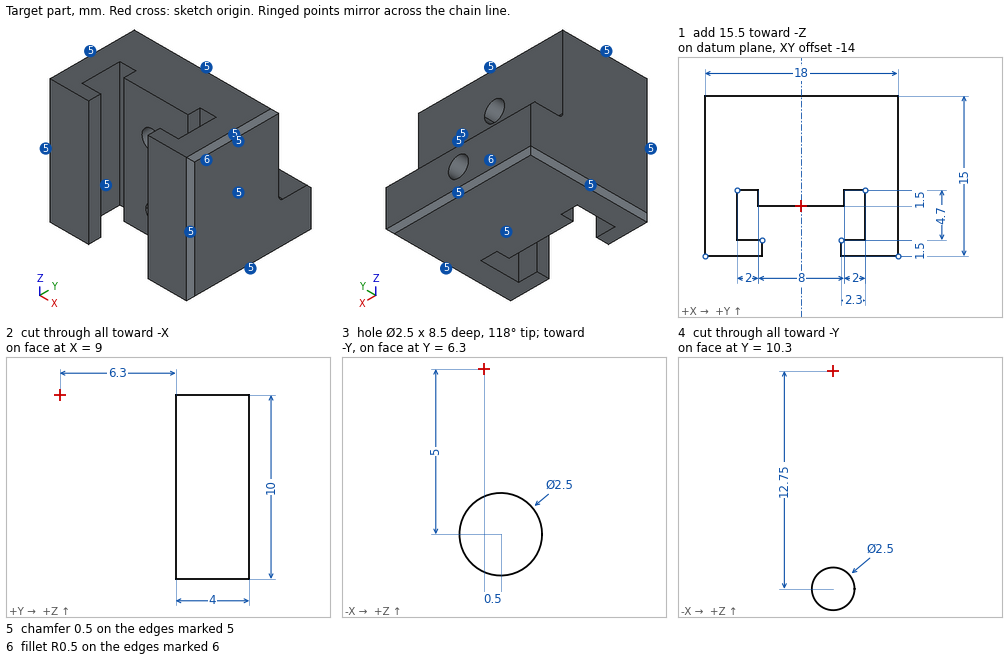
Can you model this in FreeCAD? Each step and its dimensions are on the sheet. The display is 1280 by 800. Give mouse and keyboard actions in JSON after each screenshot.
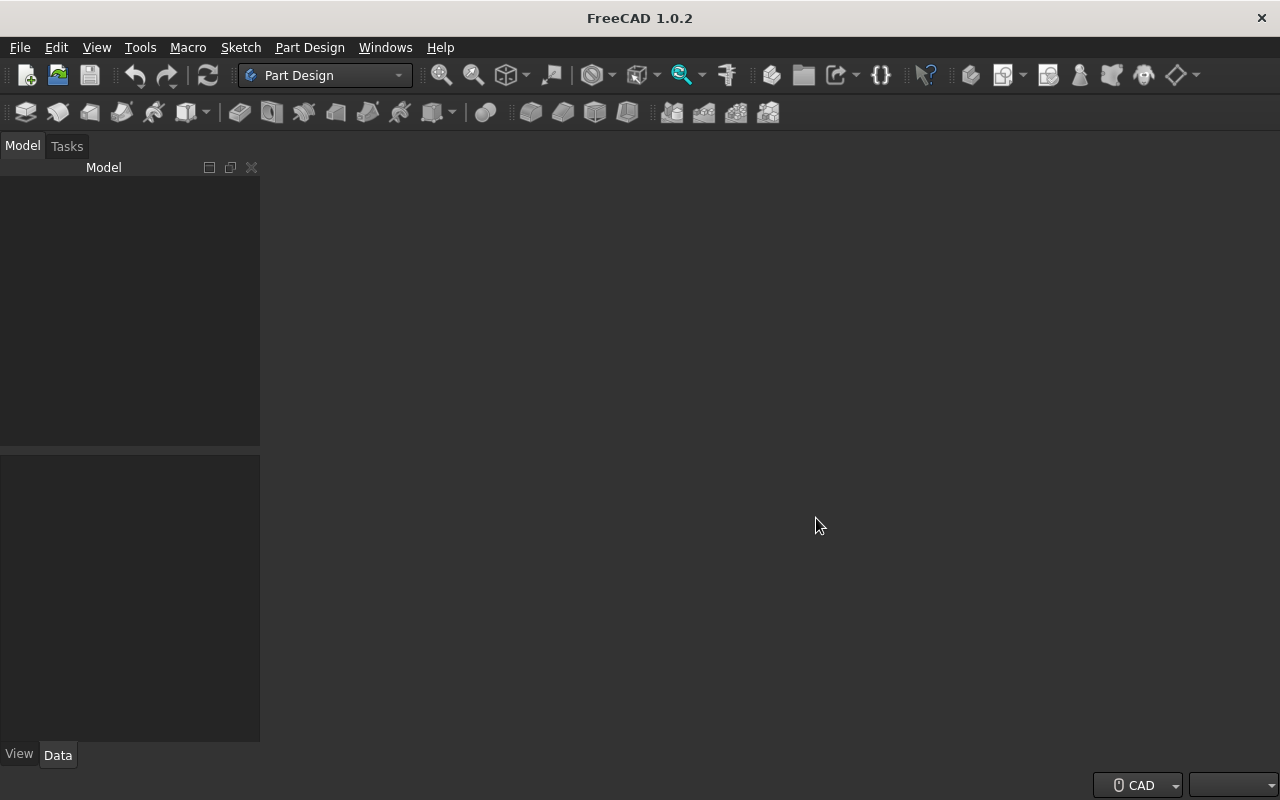
{"action": "left_click", "coordinate": [26, 76]}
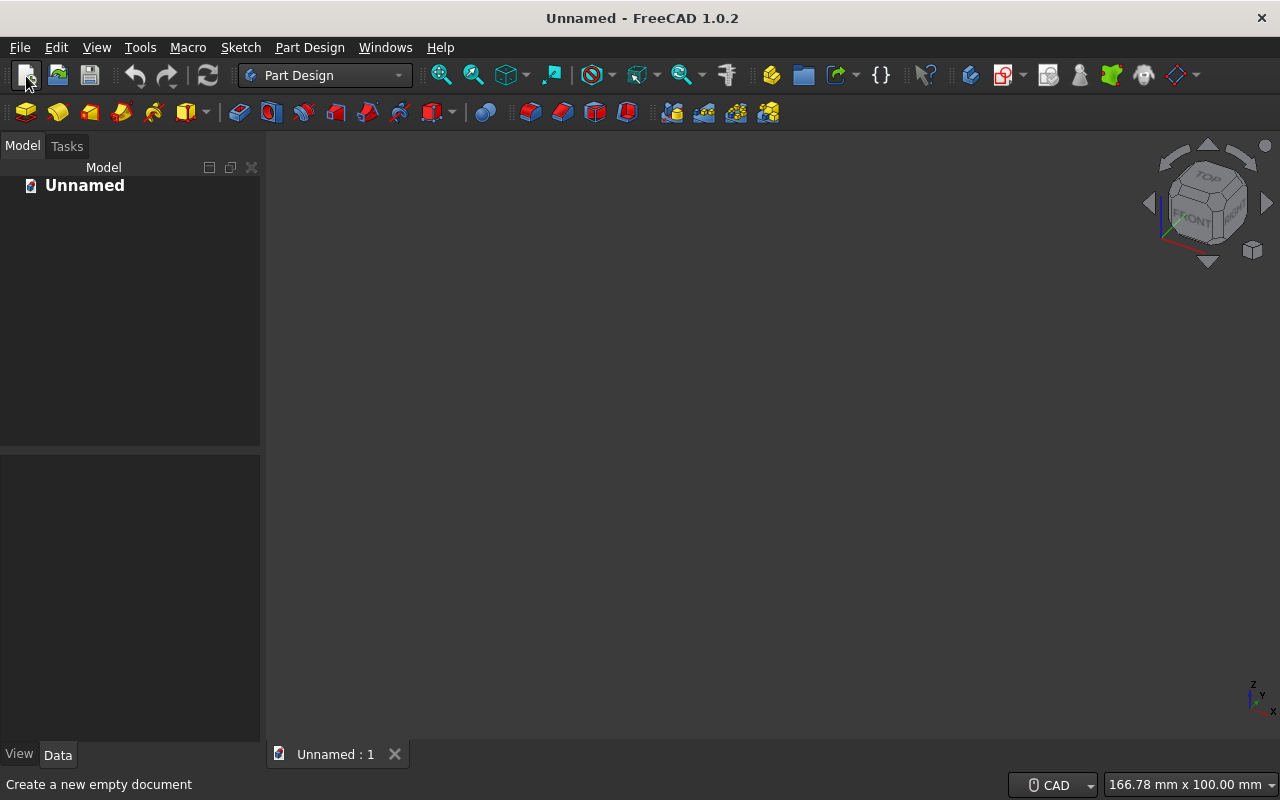
{"action": "left_click", "coordinate": [972, 76]}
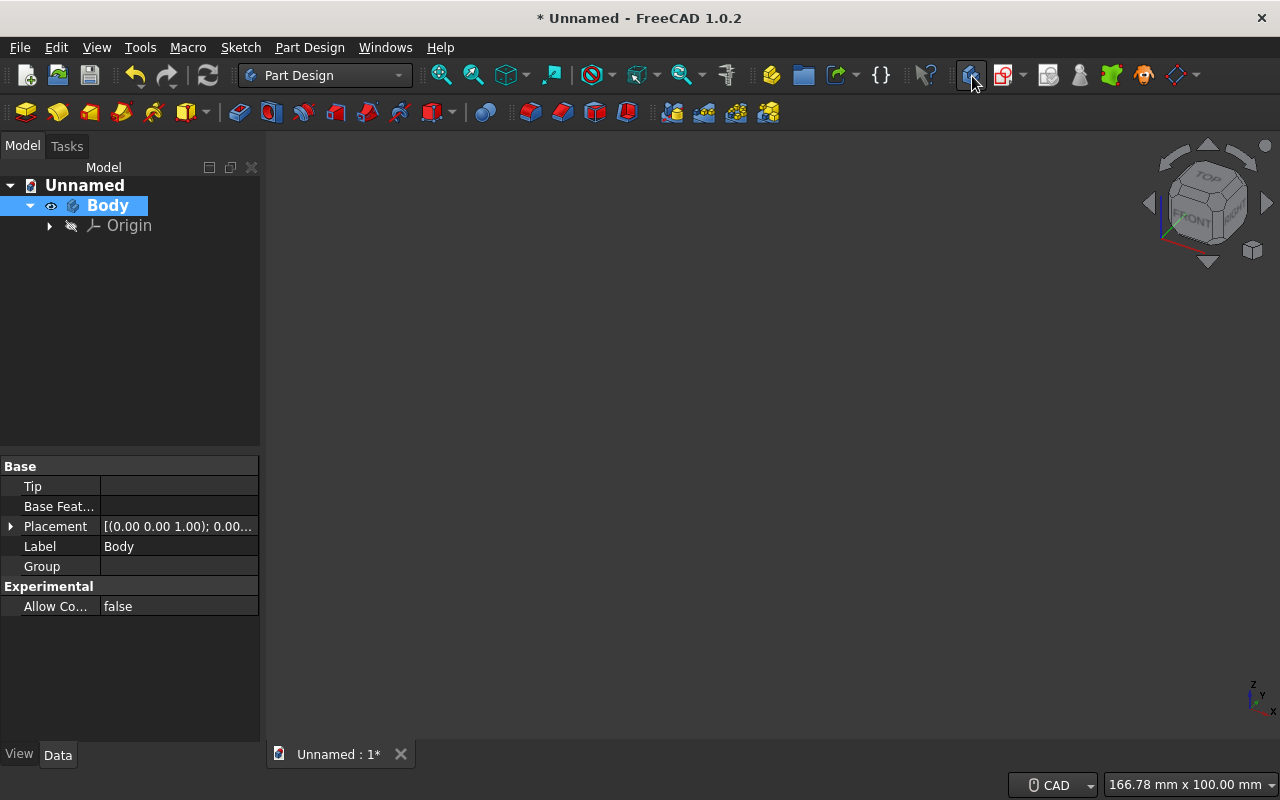
{"action": "left_click", "coordinate": [50, 226]}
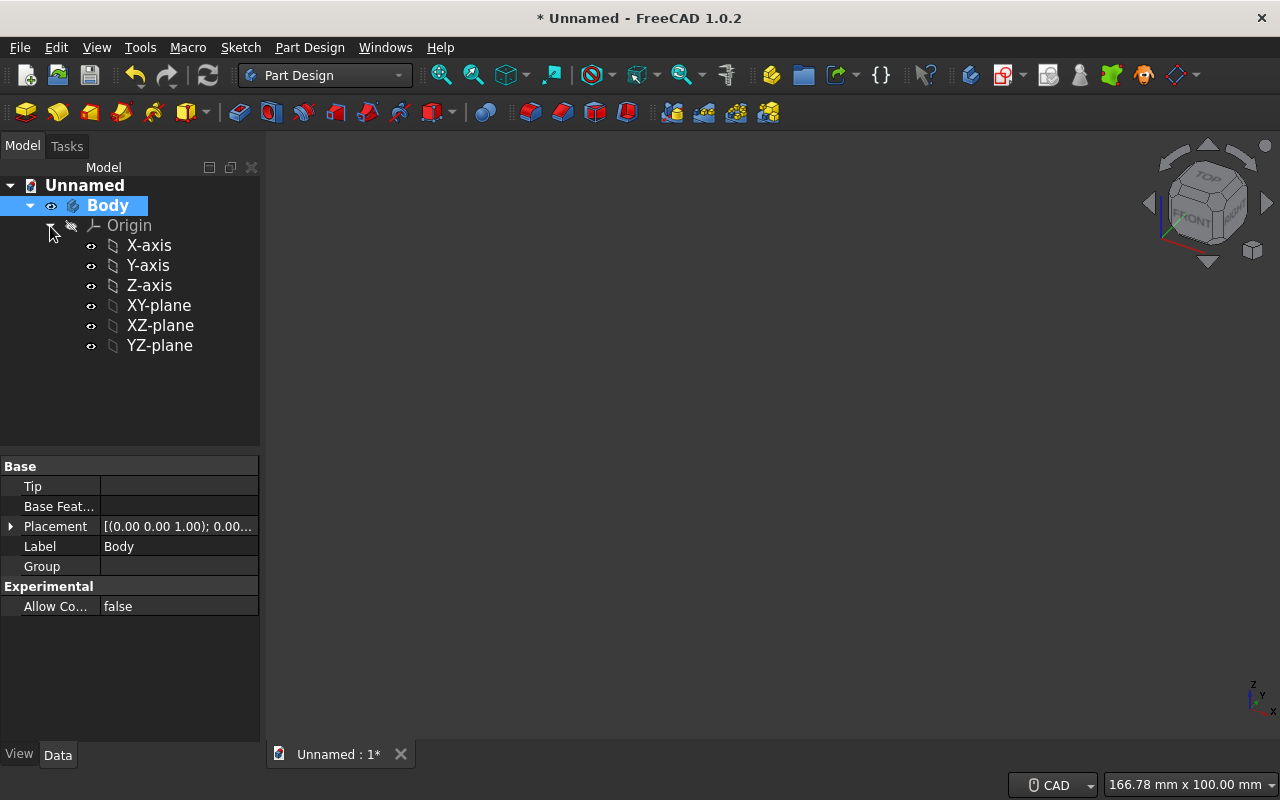
{"action": "left_click", "coordinate": [136, 306]}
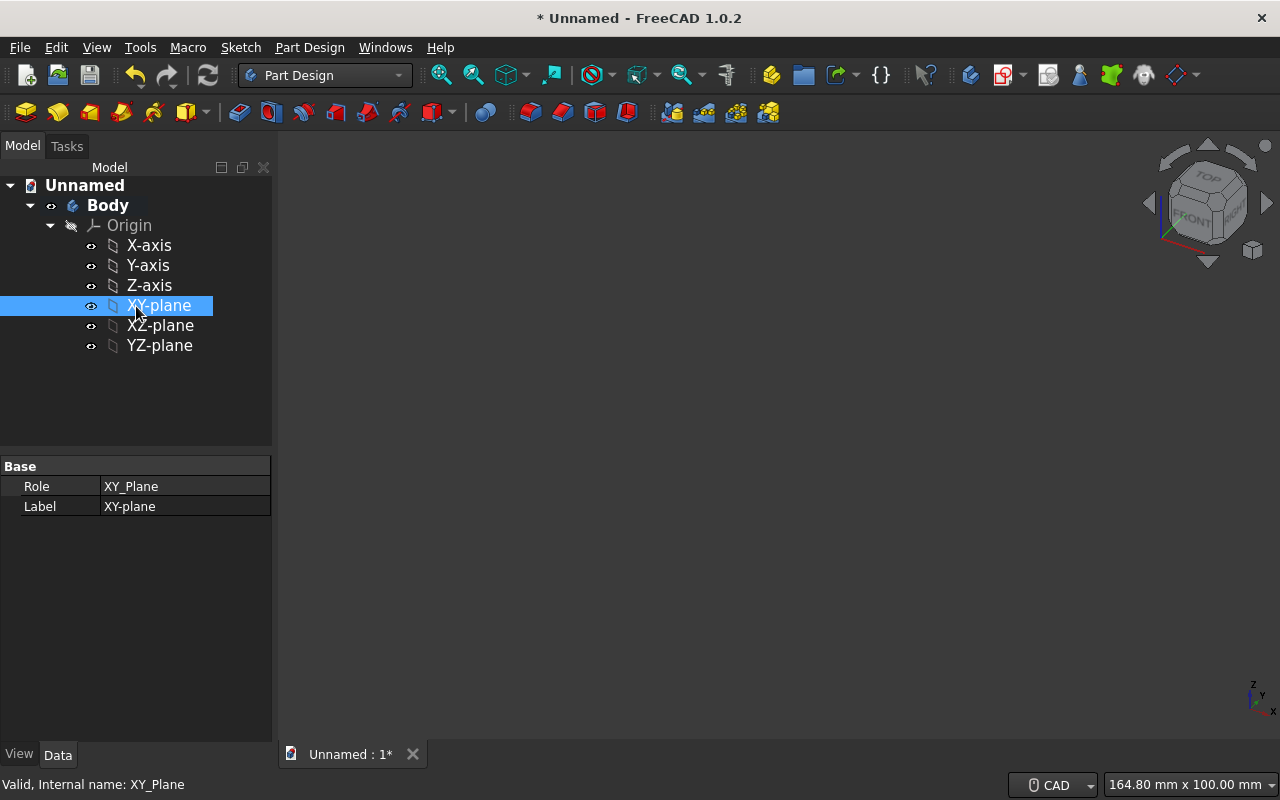
{"action": "left_click", "coordinate": [1176, 76]}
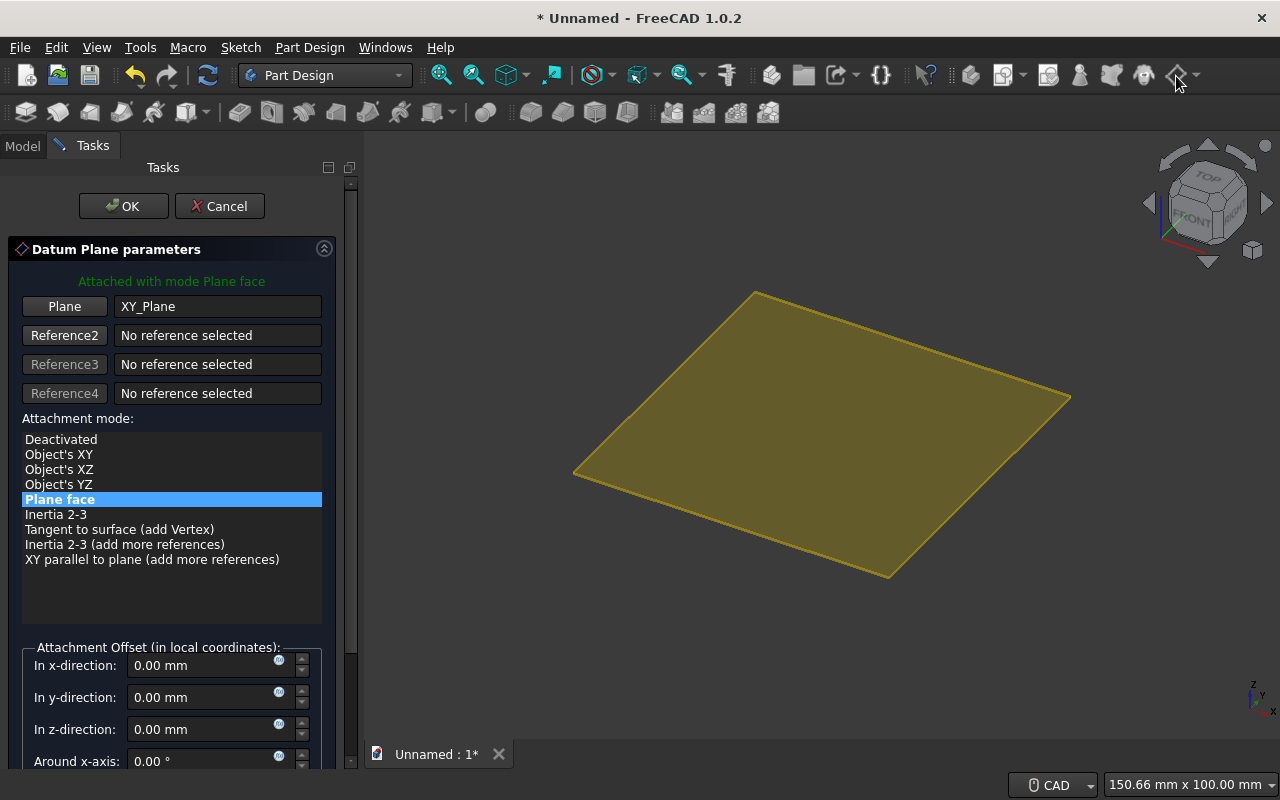
{"action": "triple_click", "coordinate": [210, 729]}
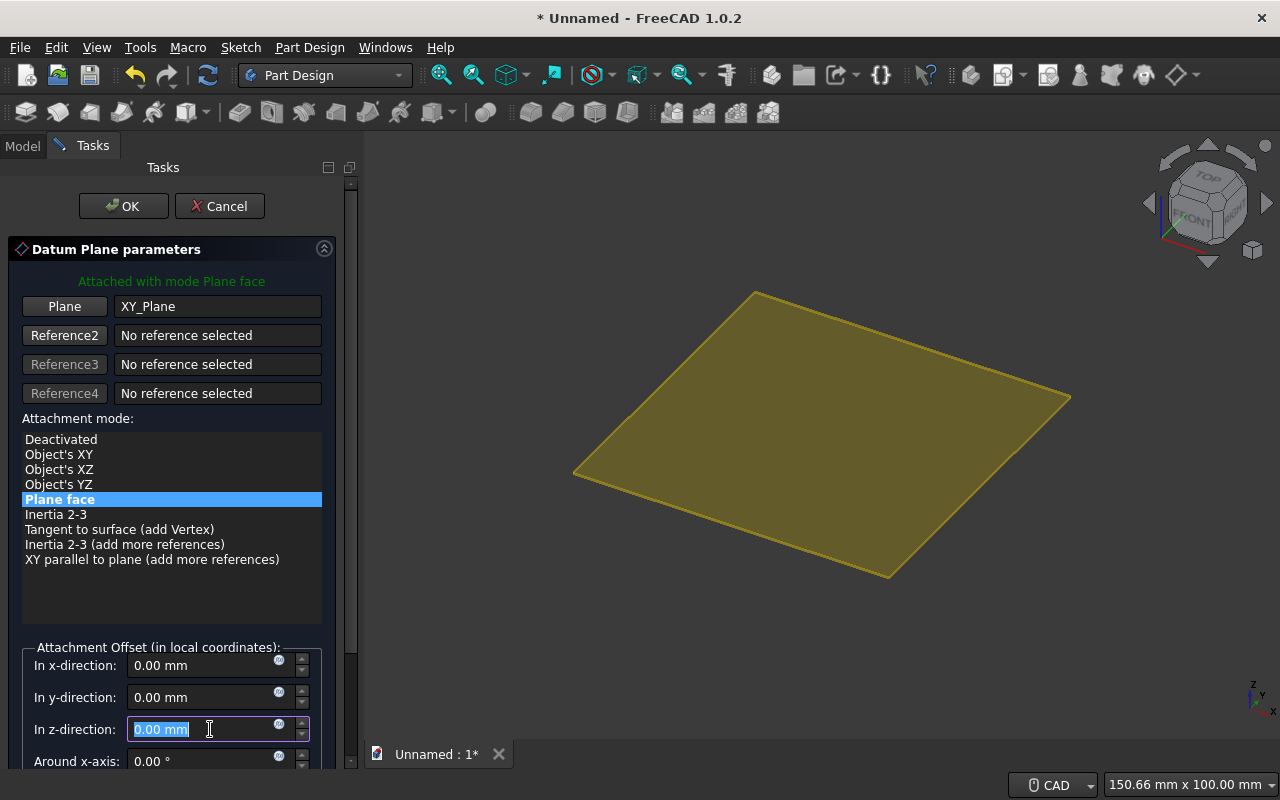
{"action": "type", "text": "-14"}
{"action": "key", "text": "Tab"}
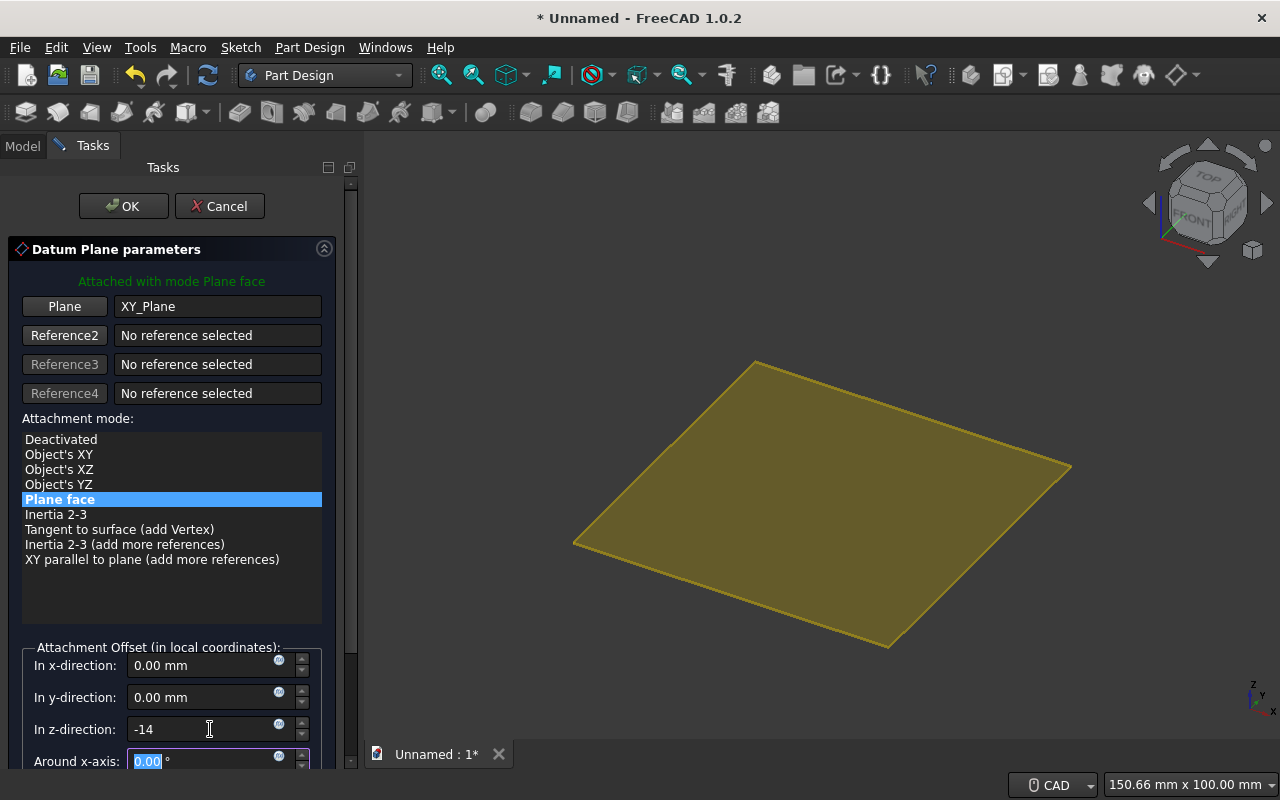
{"action": "left_click", "coordinate": [124, 206]}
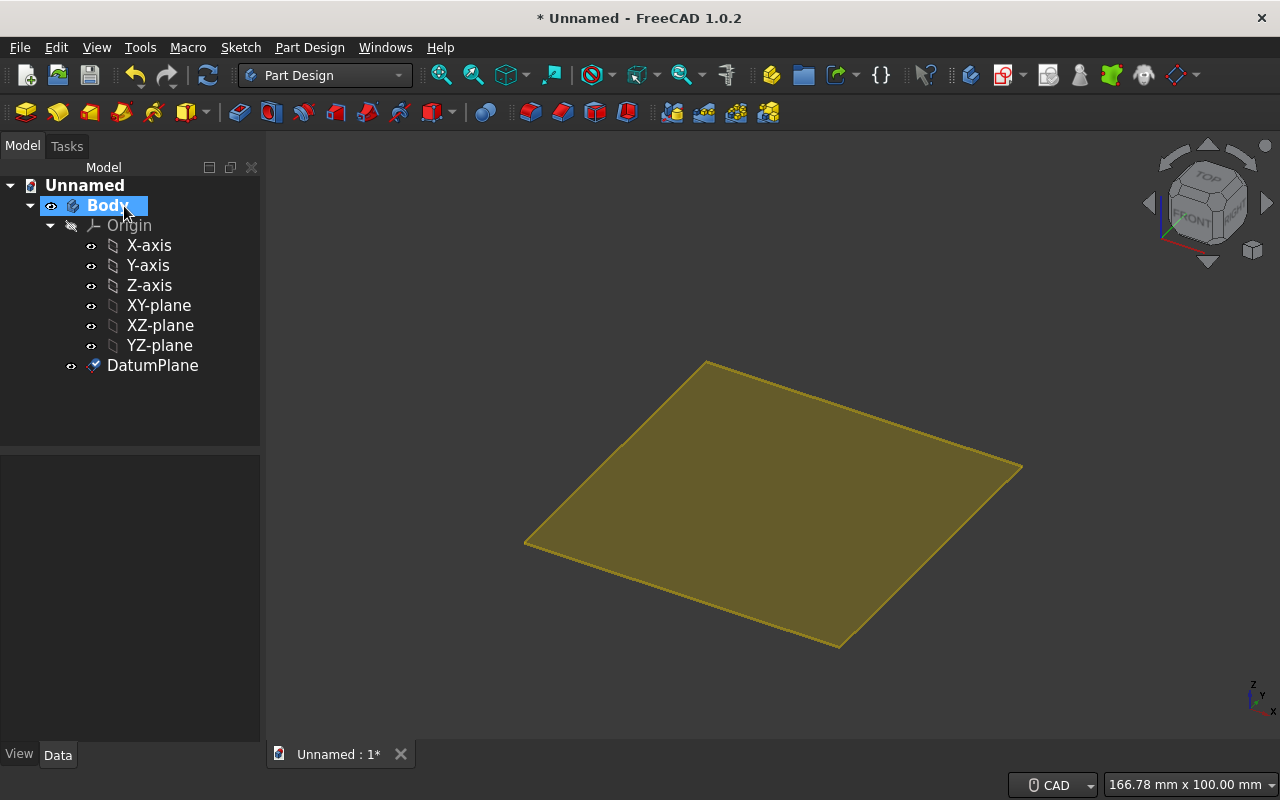
{"action": "left_click", "coordinate": [116, 366]}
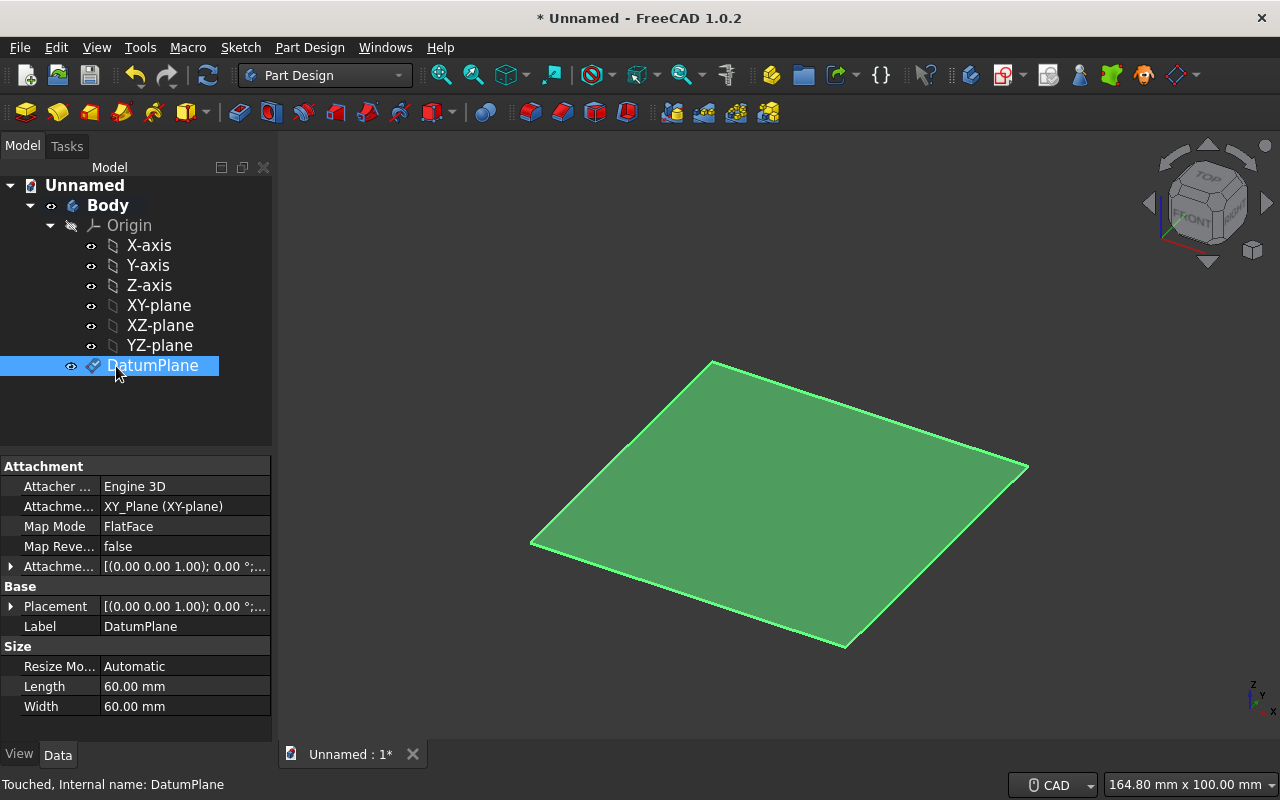
{"action": "left_click", "coordinate": [1004, 76]}